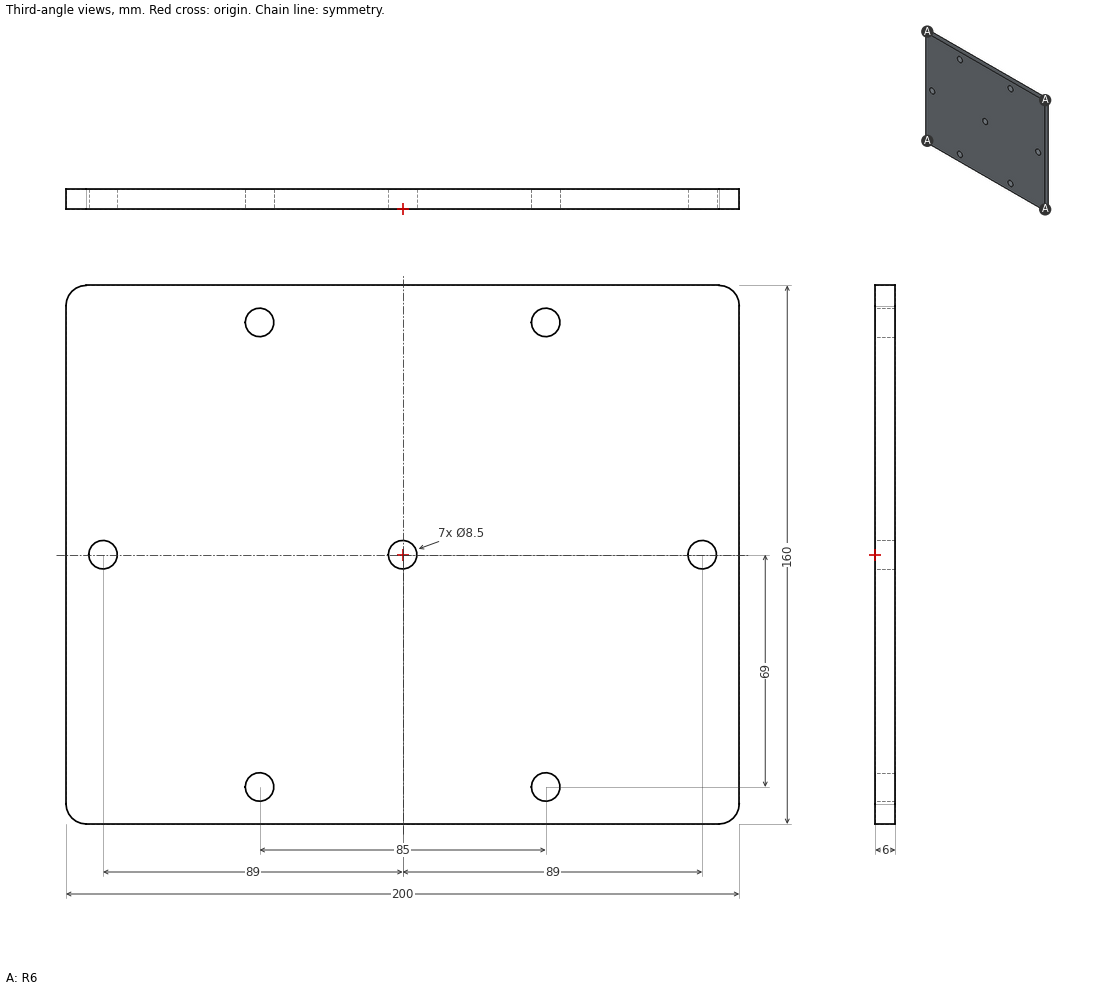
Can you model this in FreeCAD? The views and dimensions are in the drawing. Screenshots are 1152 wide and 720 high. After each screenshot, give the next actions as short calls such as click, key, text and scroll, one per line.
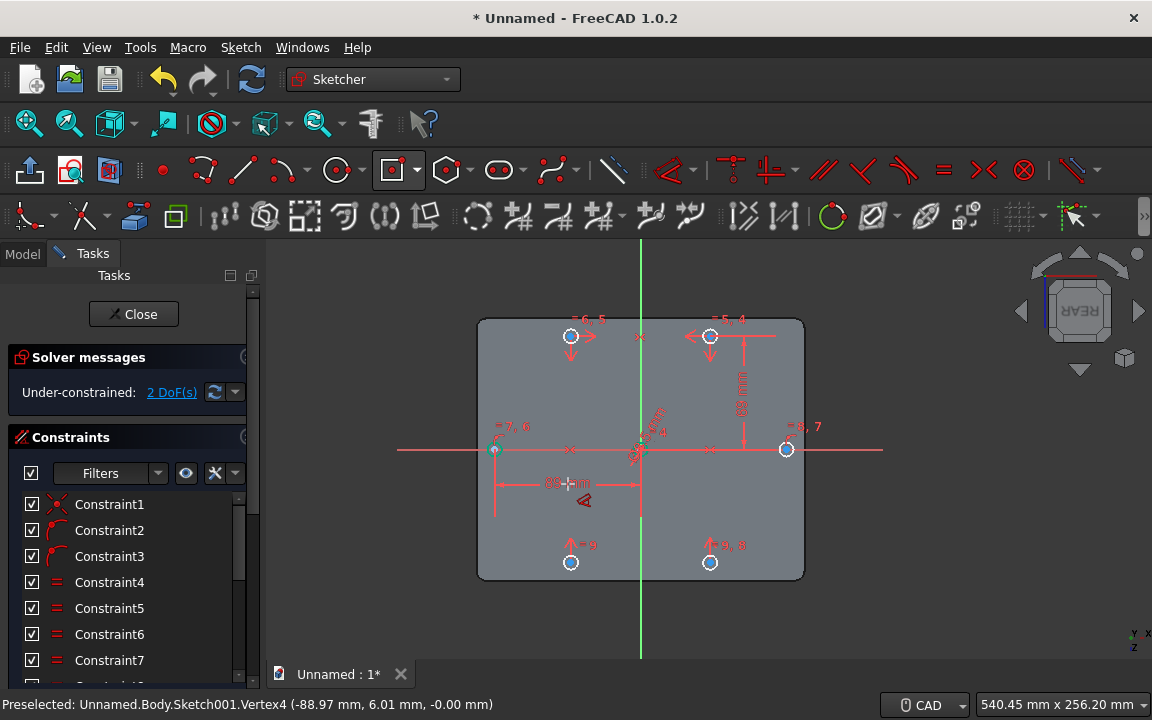
click(787, 450)
click(714, 484)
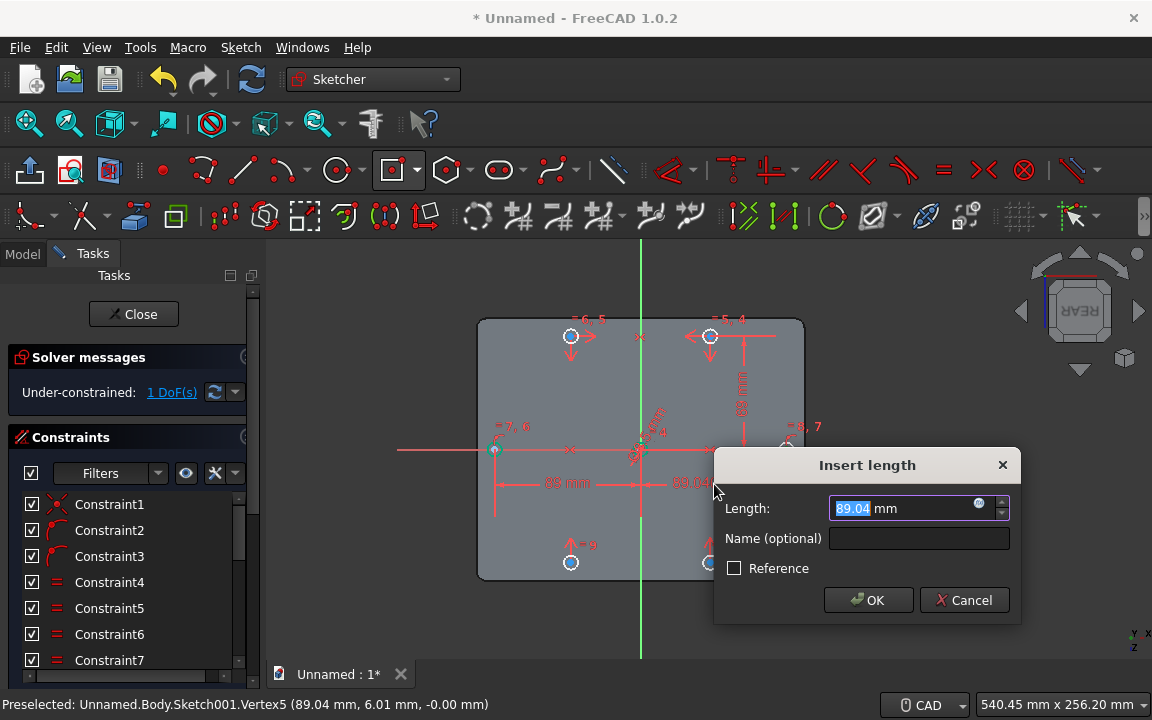
text(89)
key(Return)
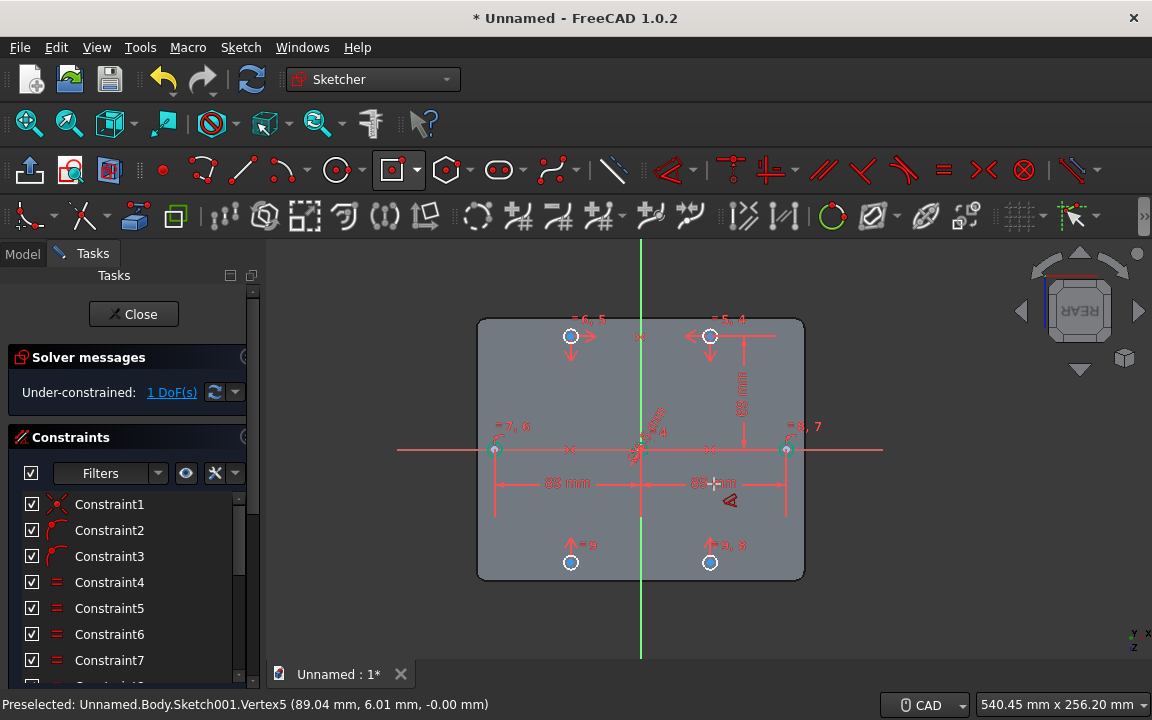
click(710, 336)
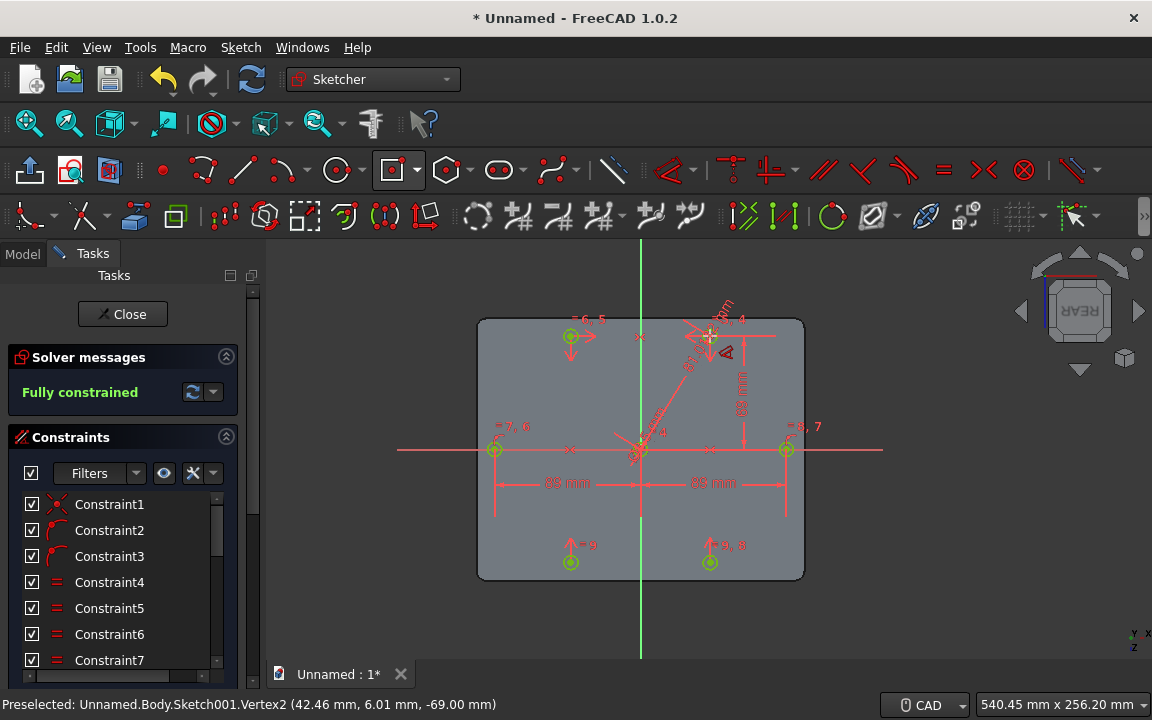
click(571, 336)
click(609, 302)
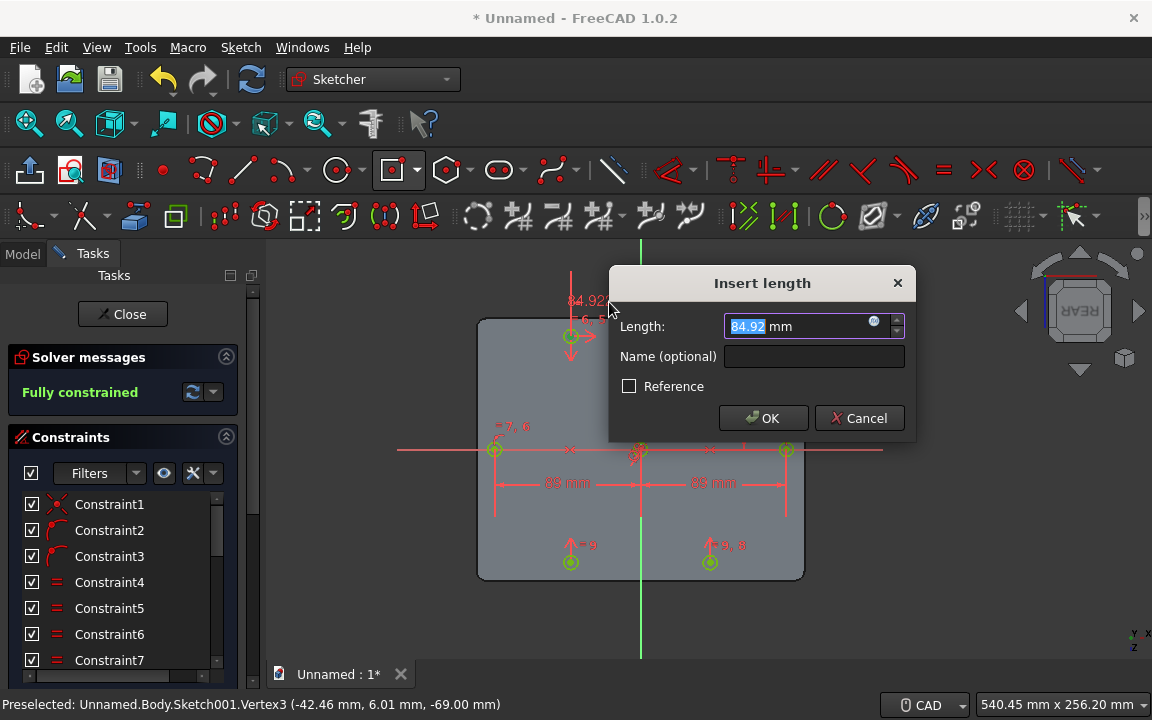
text(85)
key(Return)
key(Escape)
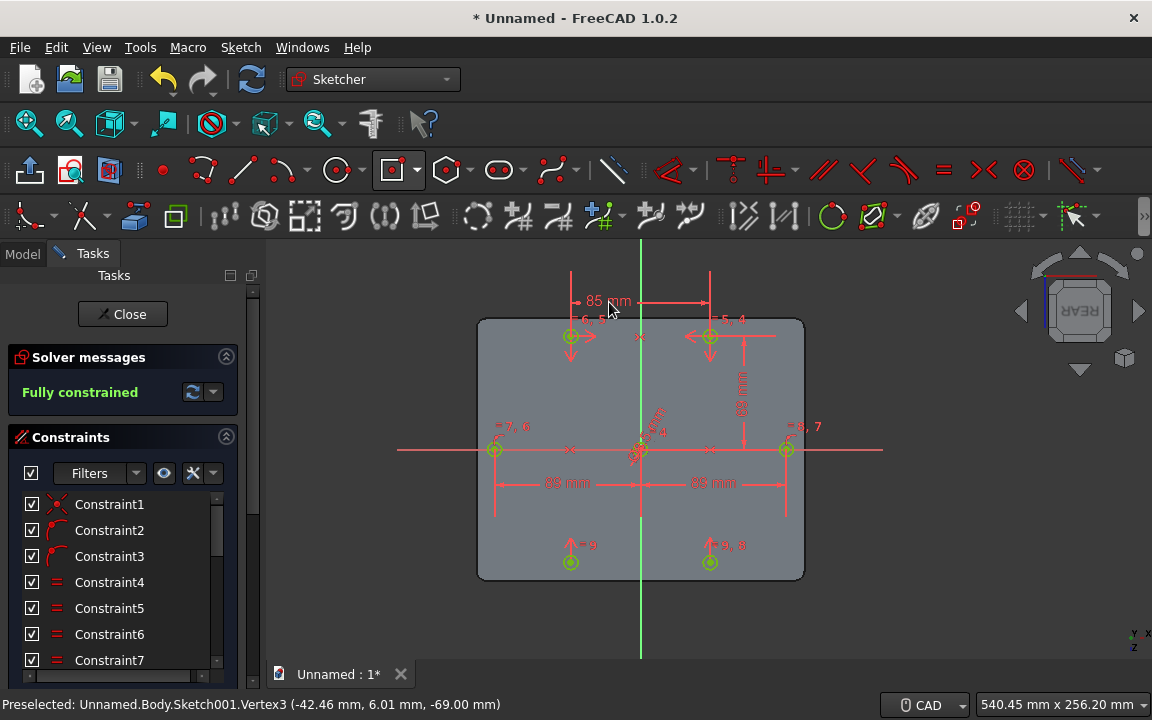
click(123, 314)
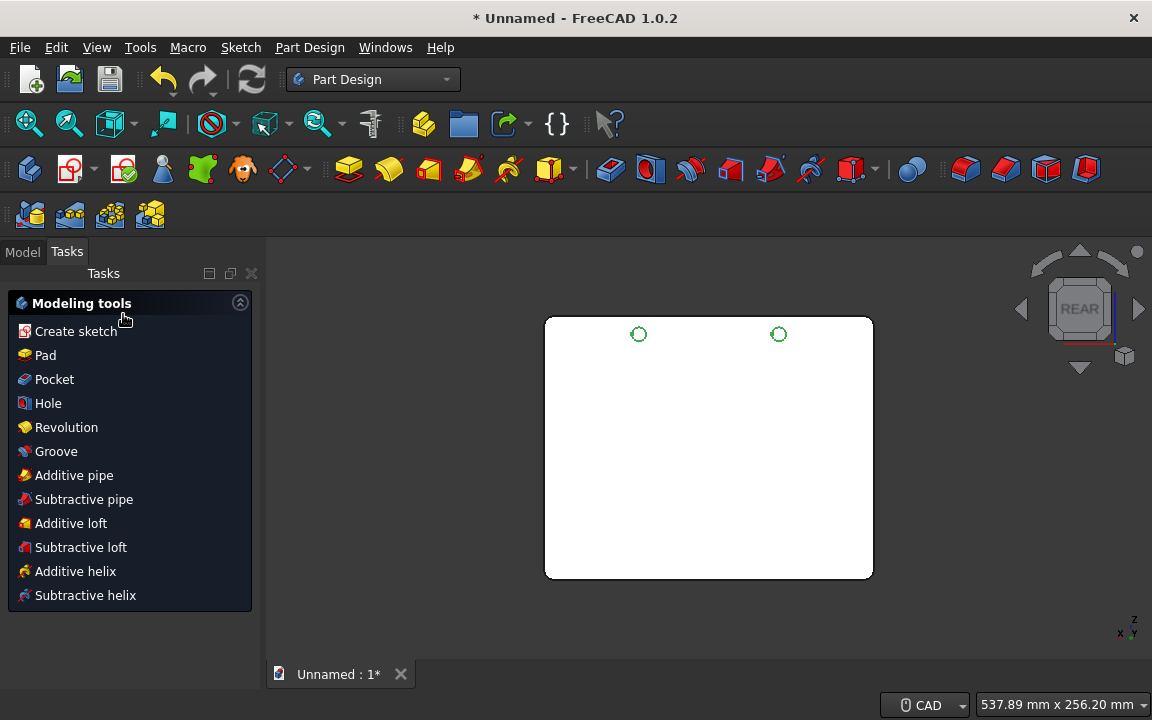
click(612, 170)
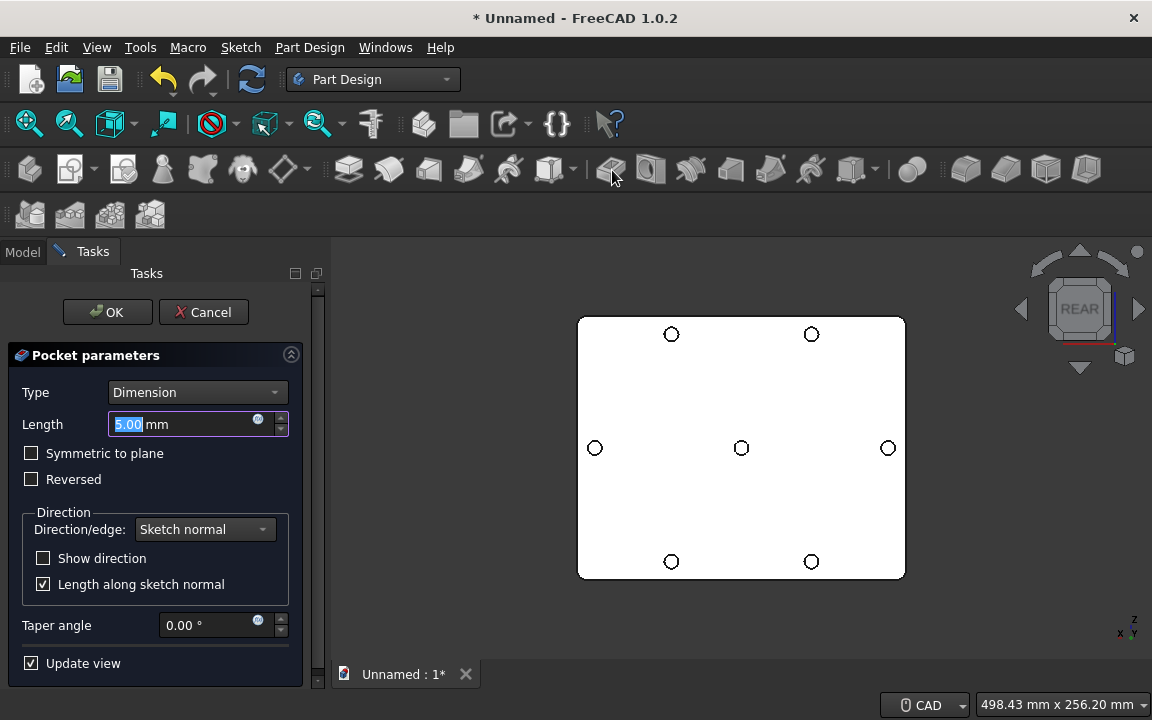
click(198, 392)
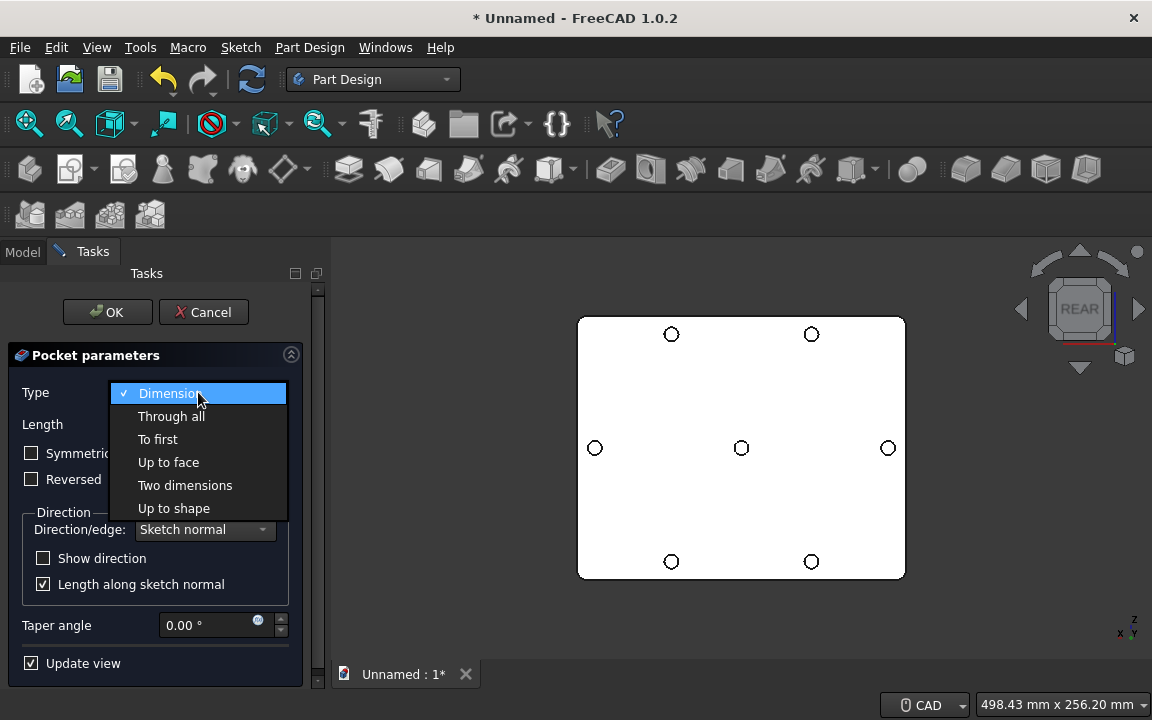
click(198, 416)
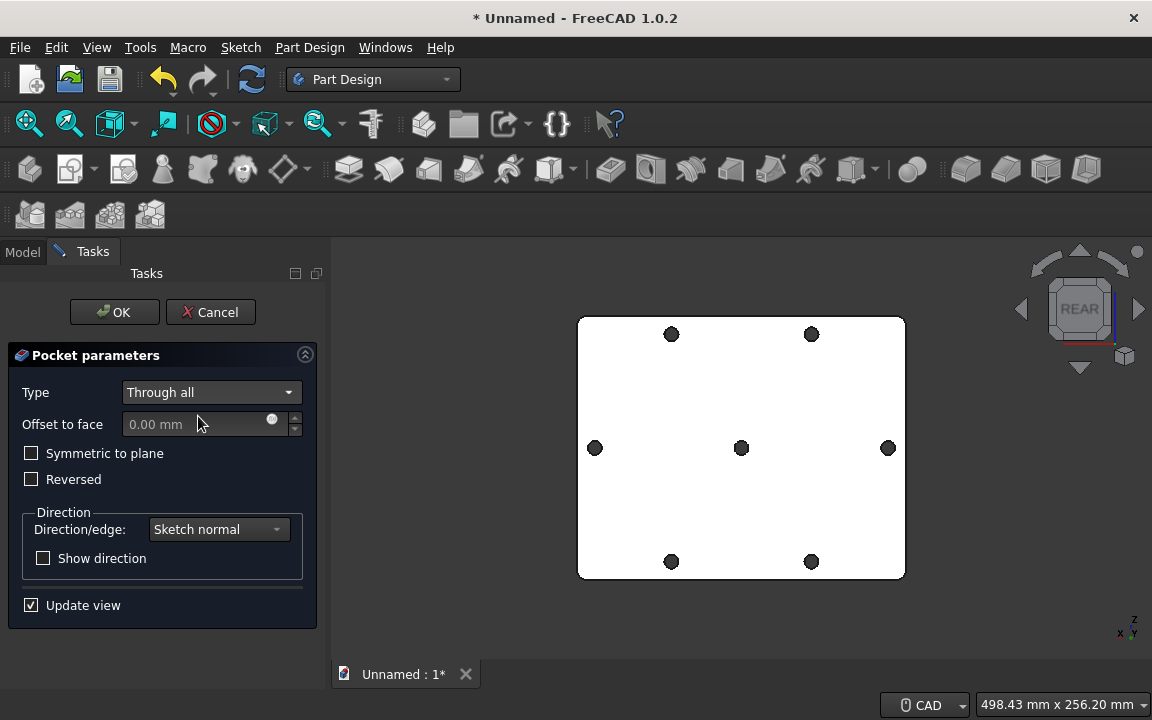
click(115, 312)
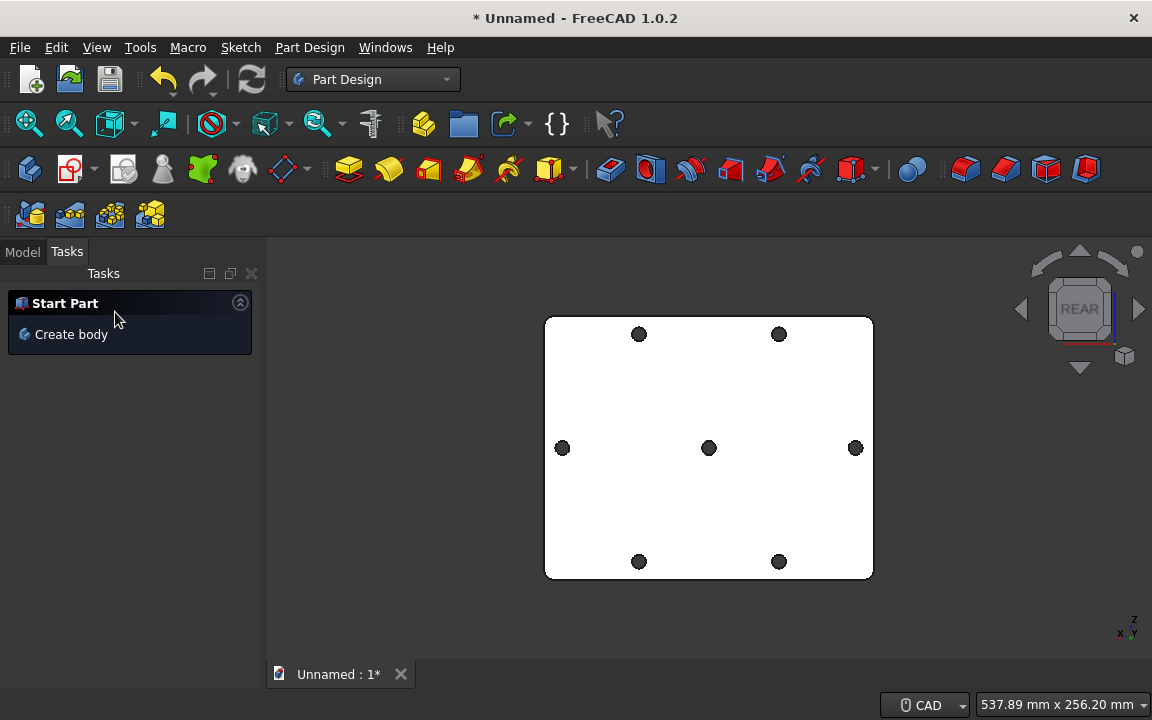
key(0)